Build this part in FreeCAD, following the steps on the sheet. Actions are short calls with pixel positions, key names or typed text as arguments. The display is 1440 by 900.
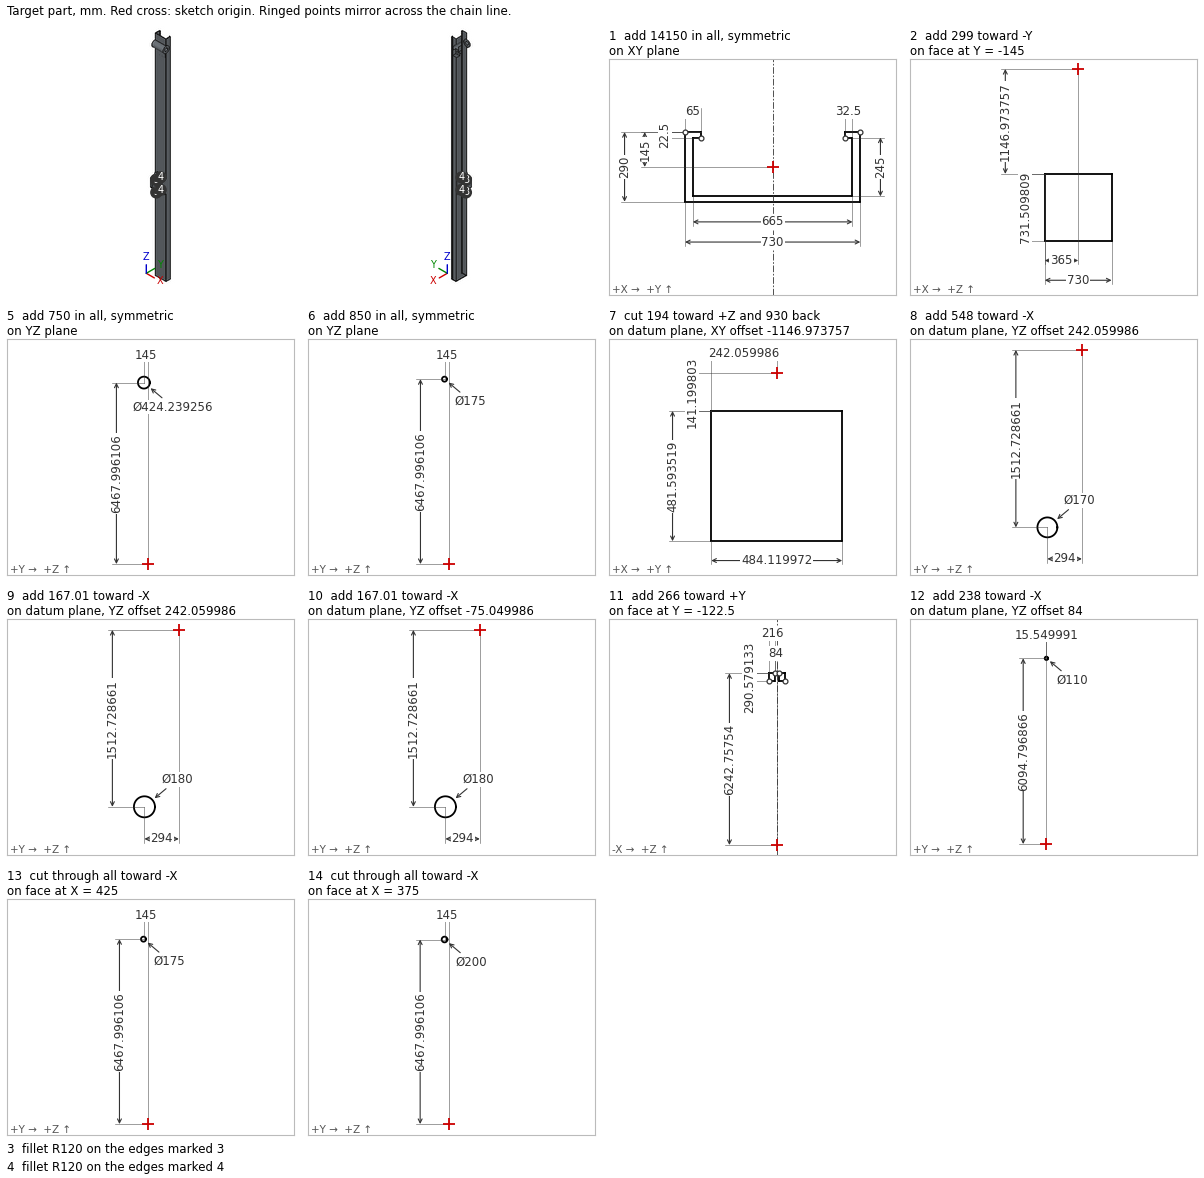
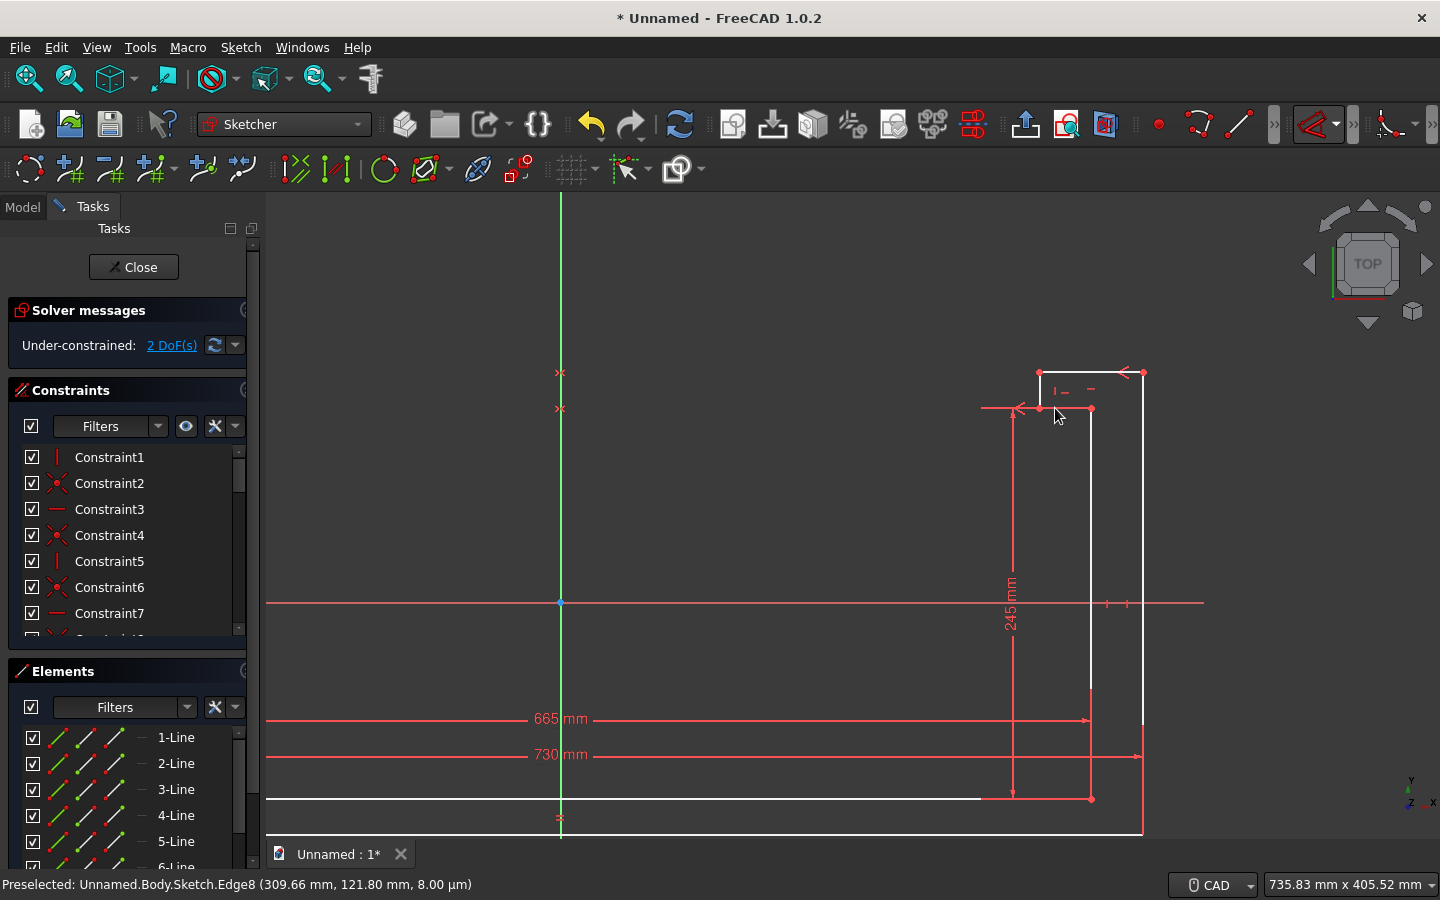
key(l)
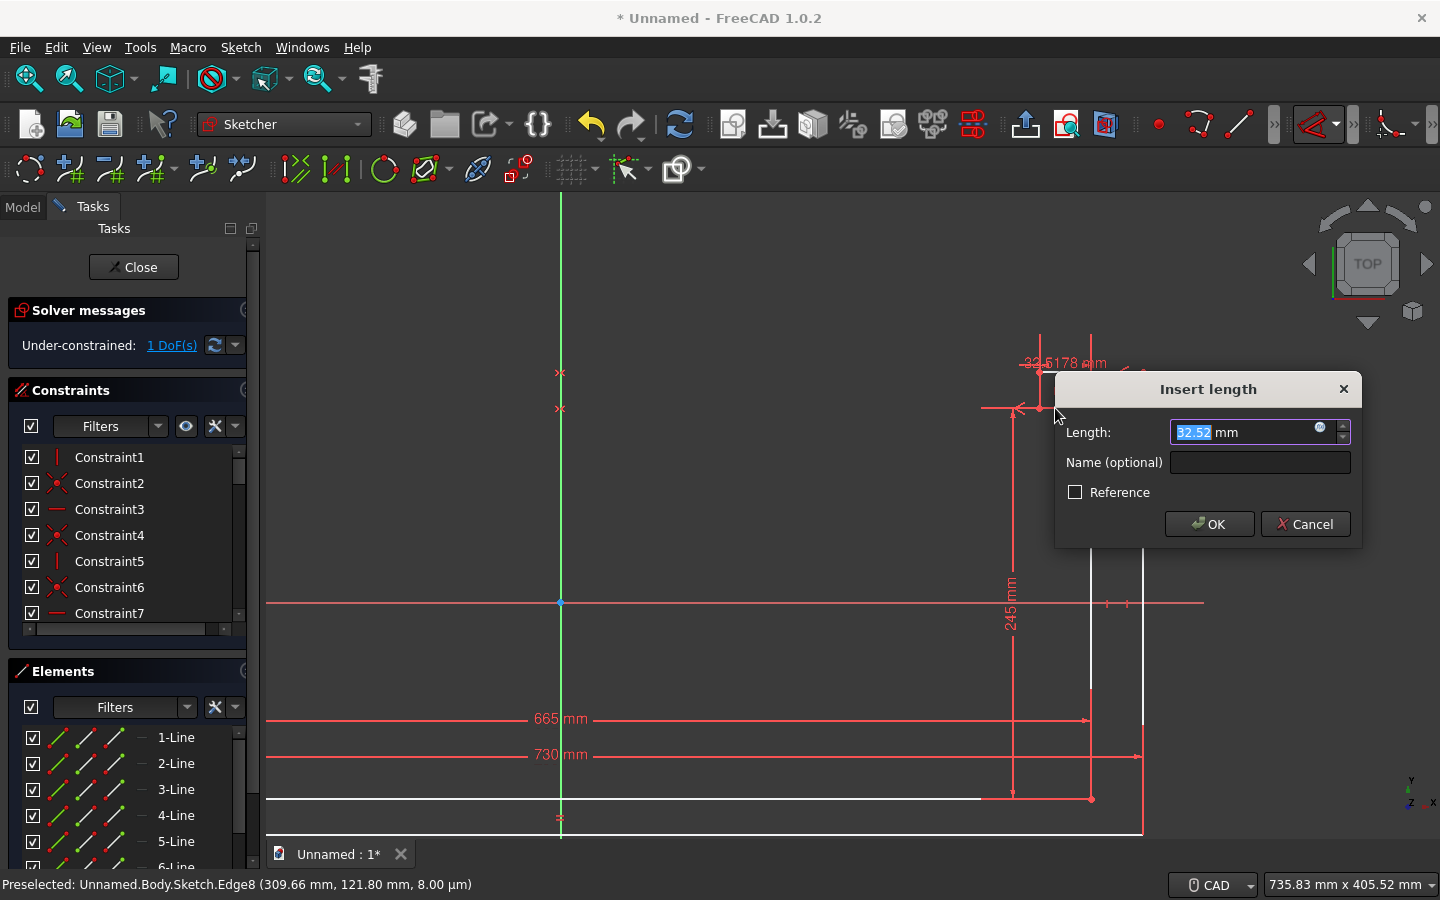
text(32.5)
key(Return)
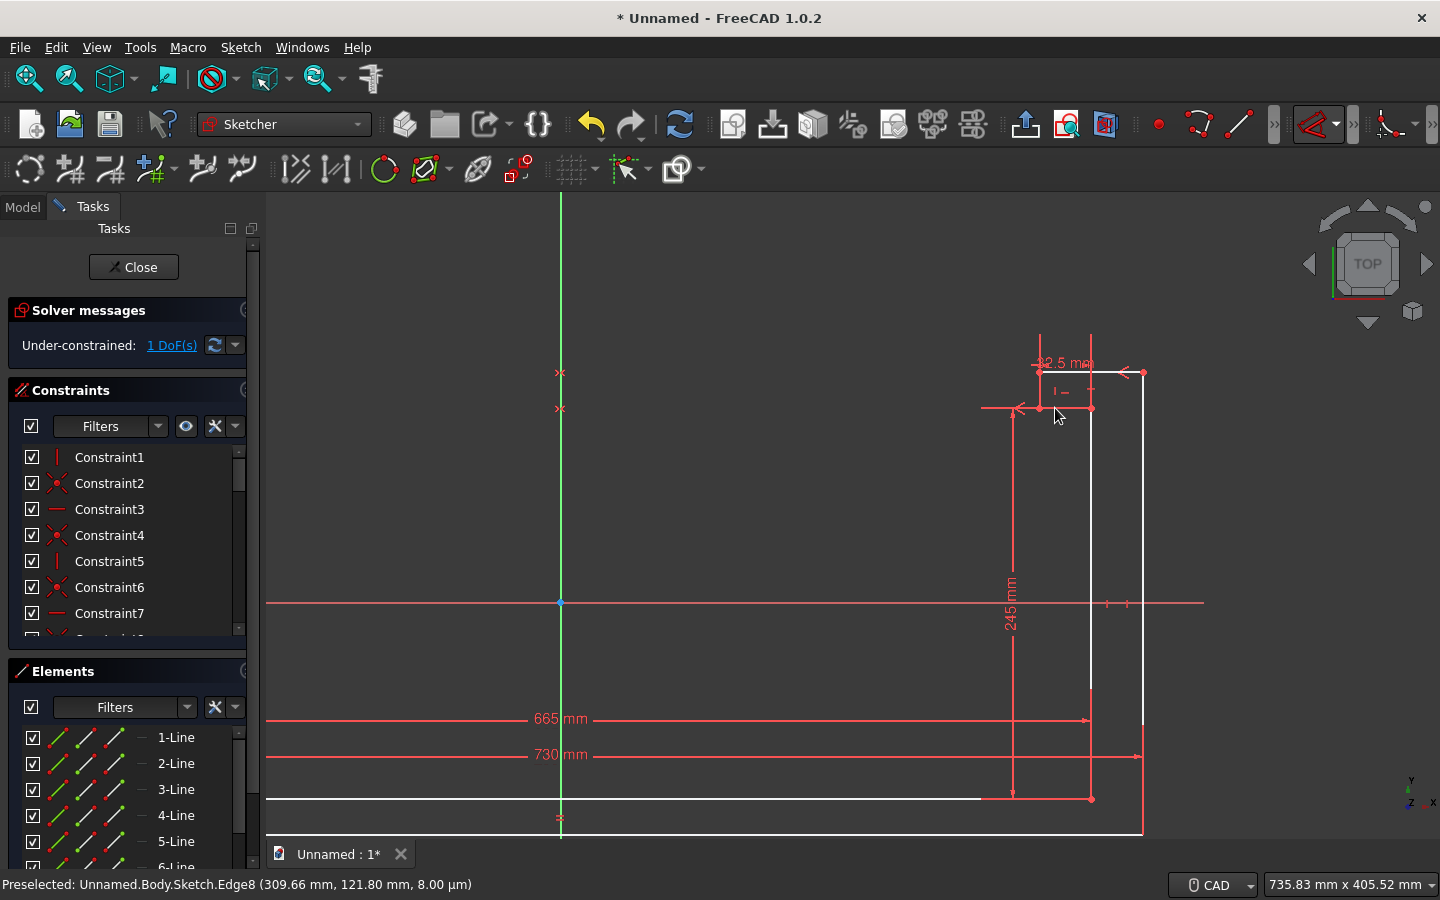
scroll(1056, 409, down, 3)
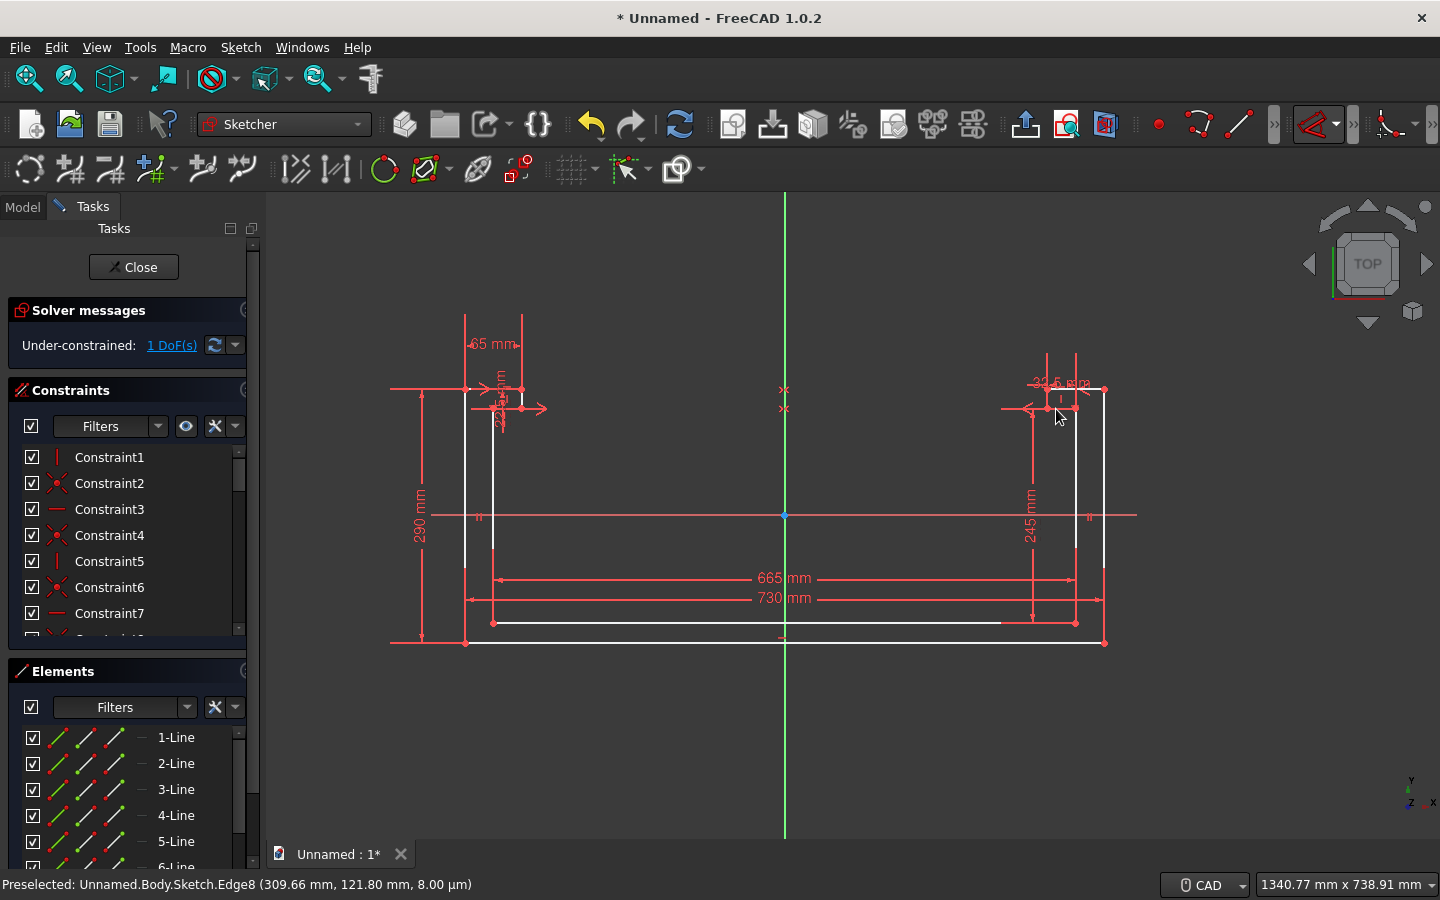
click(522, 389)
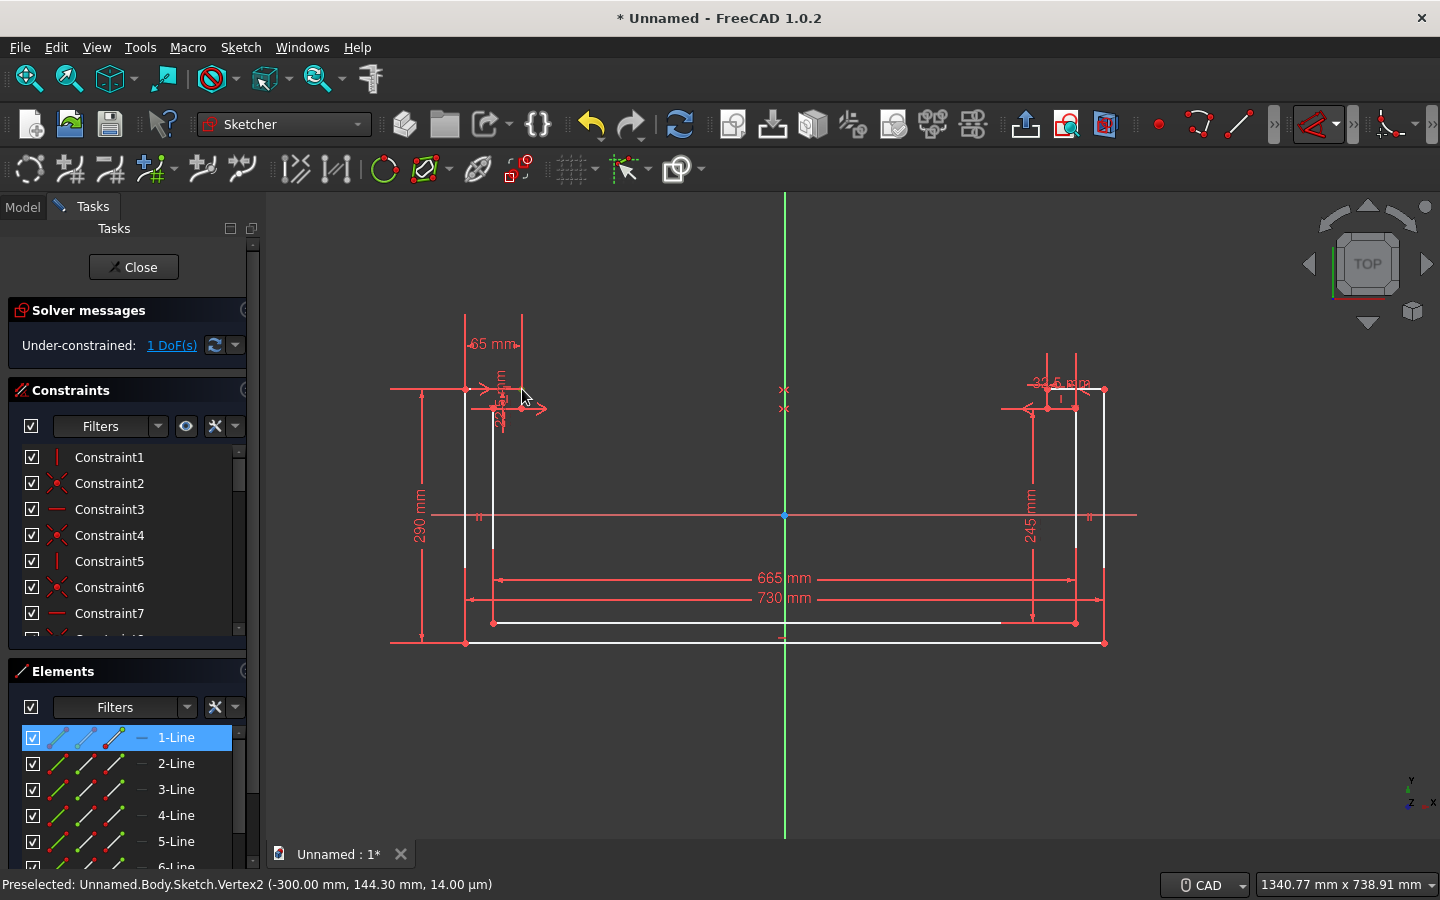
click(1338, 124)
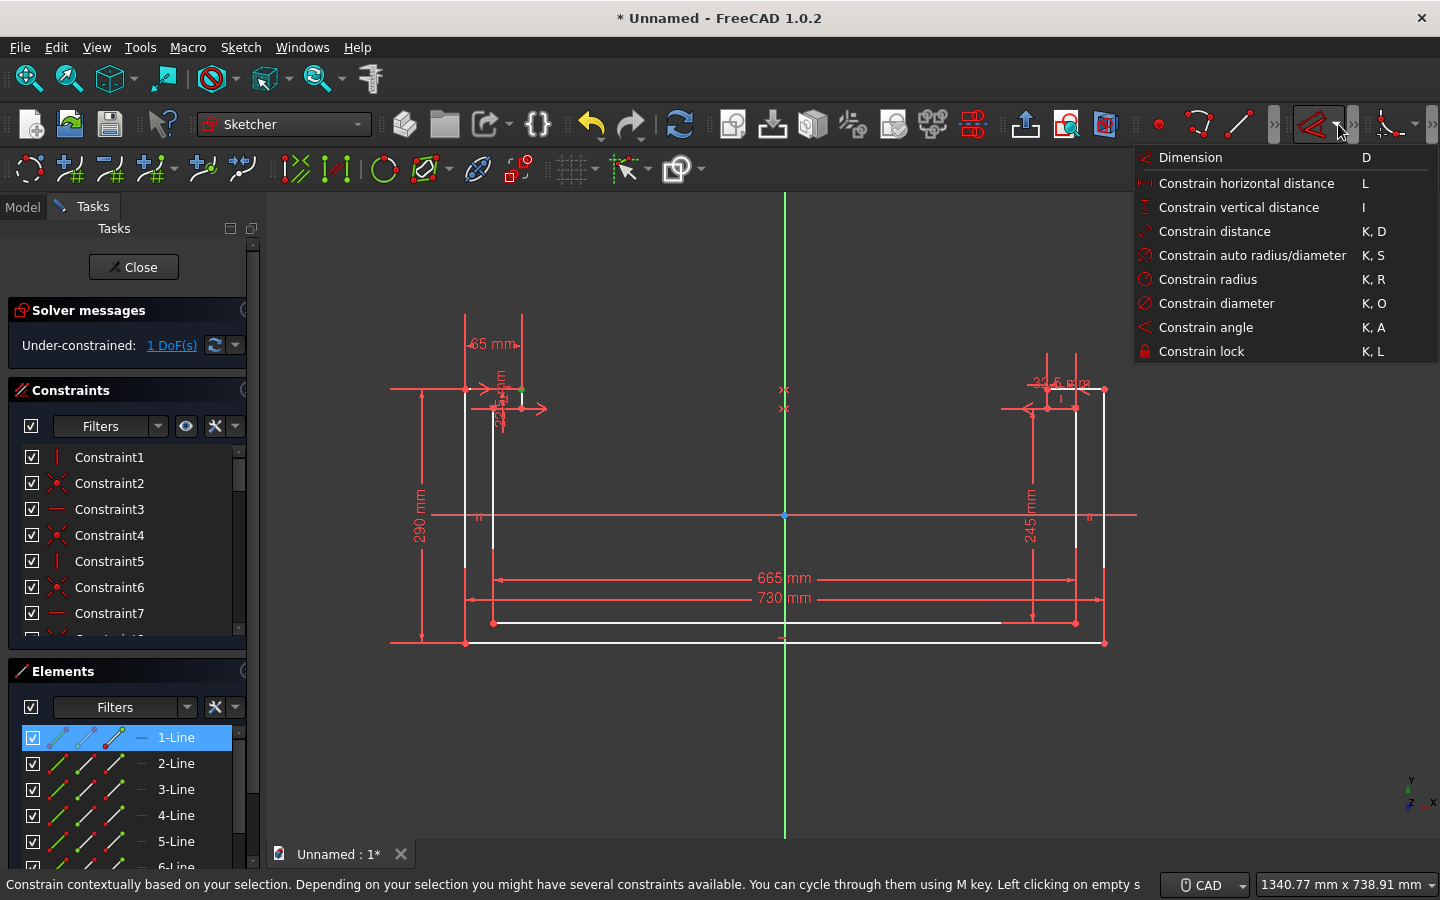
click(1286, 207)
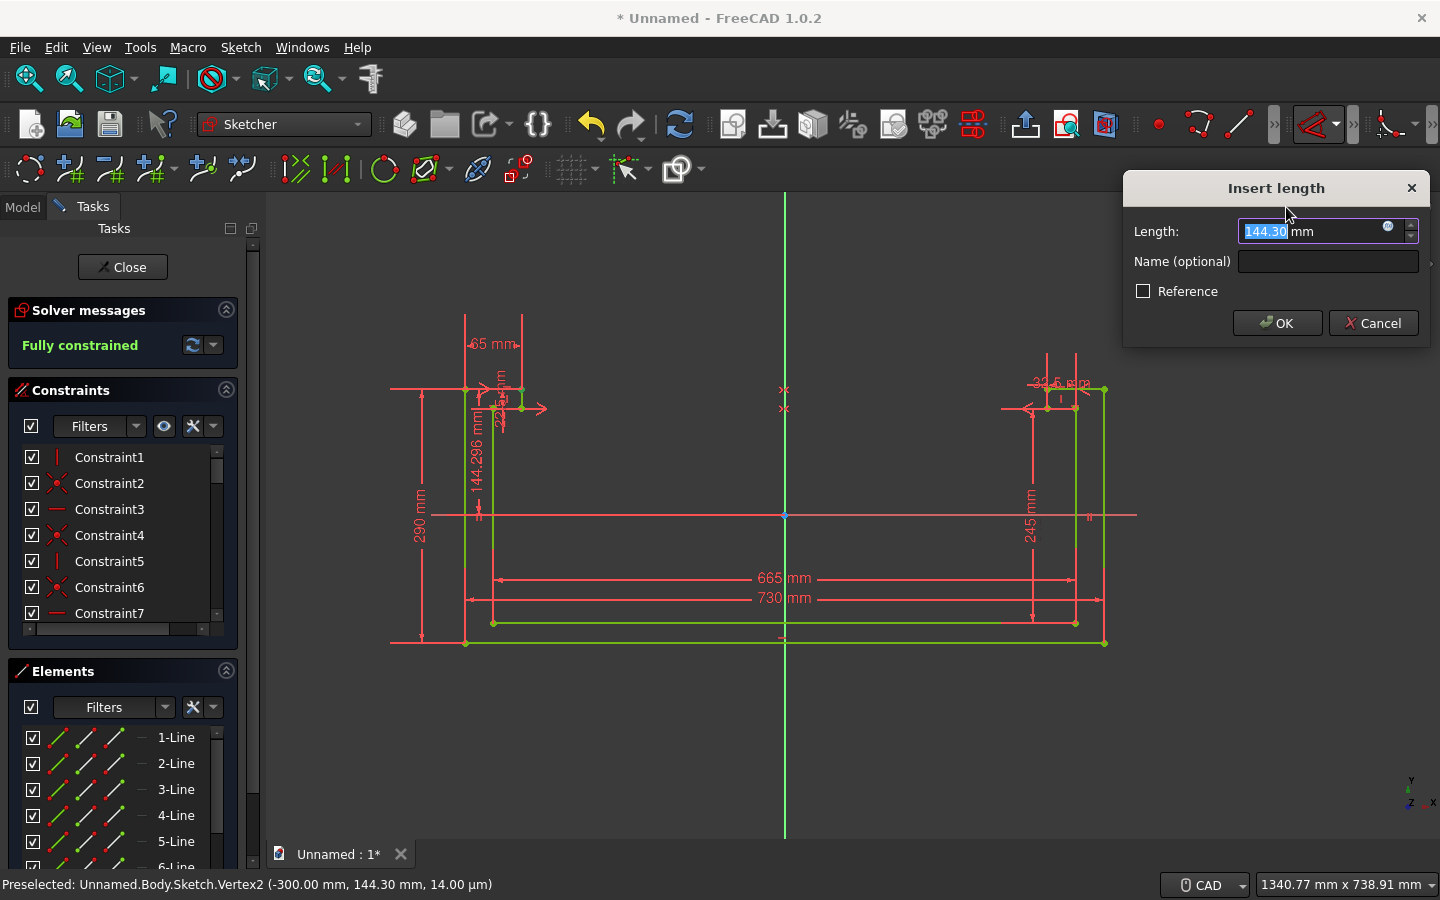
text(145)
key(Return)